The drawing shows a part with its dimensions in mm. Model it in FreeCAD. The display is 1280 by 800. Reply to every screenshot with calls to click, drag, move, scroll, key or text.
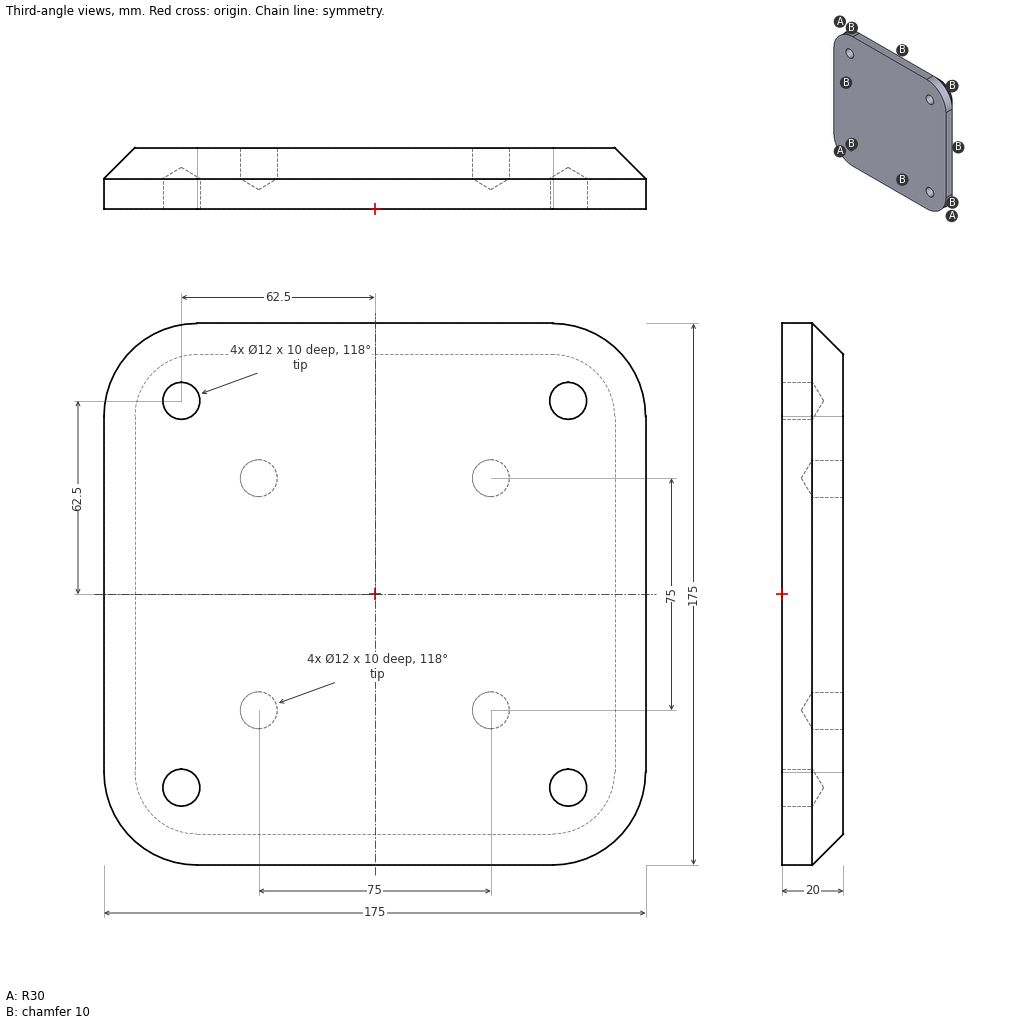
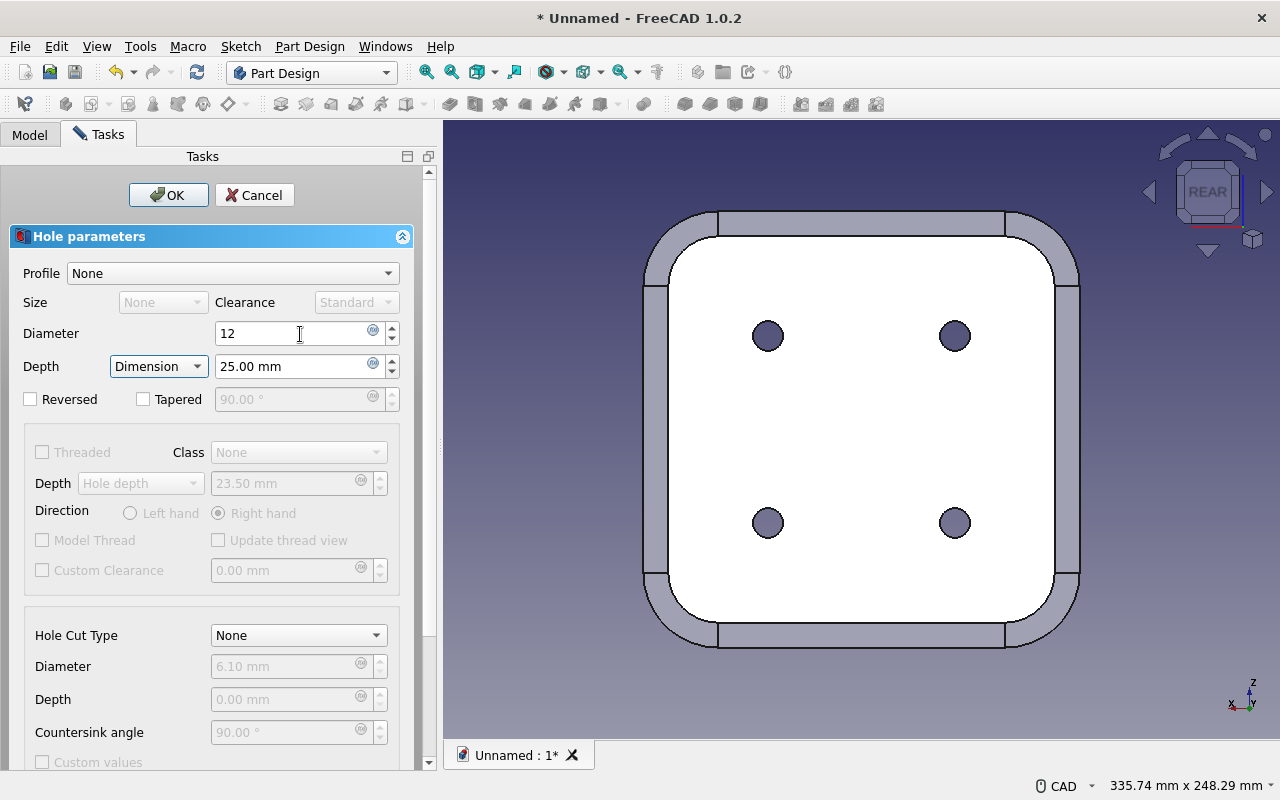
triple_click(300, 366)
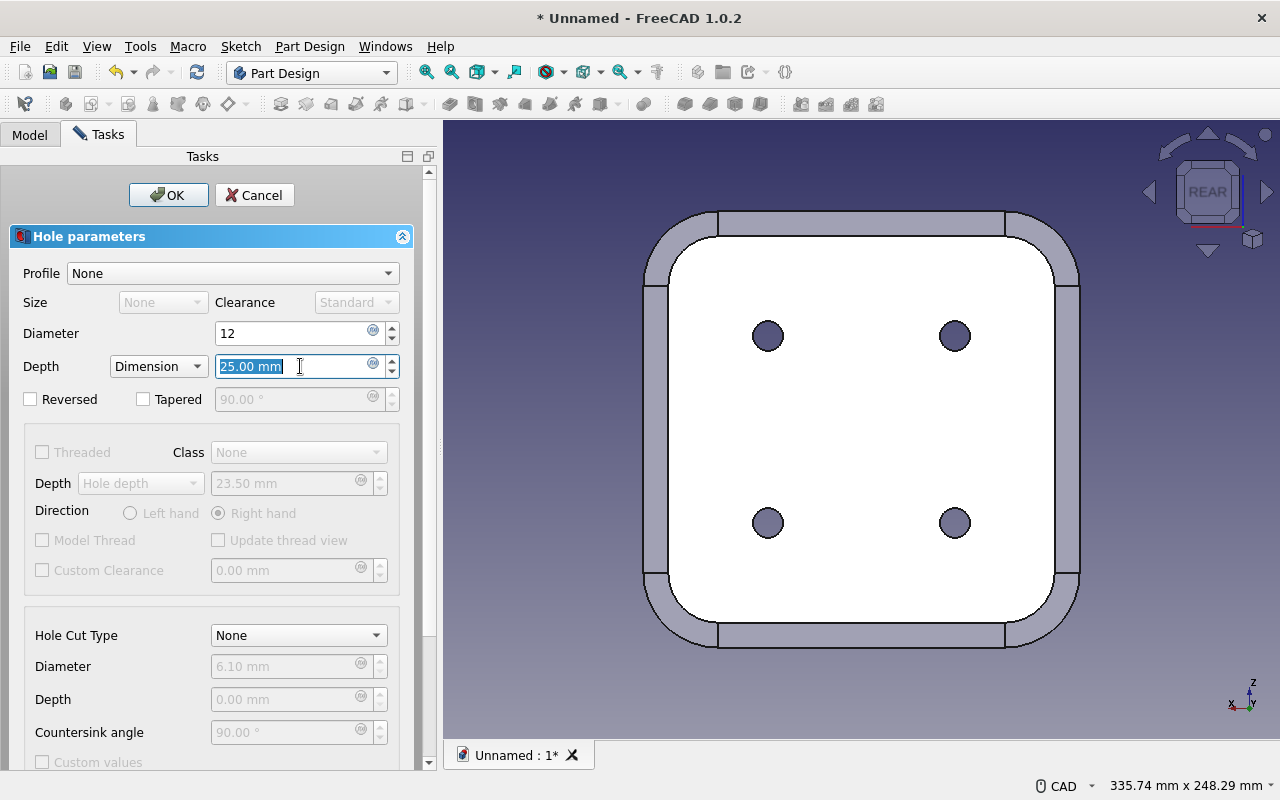
text(10)
key(Tab)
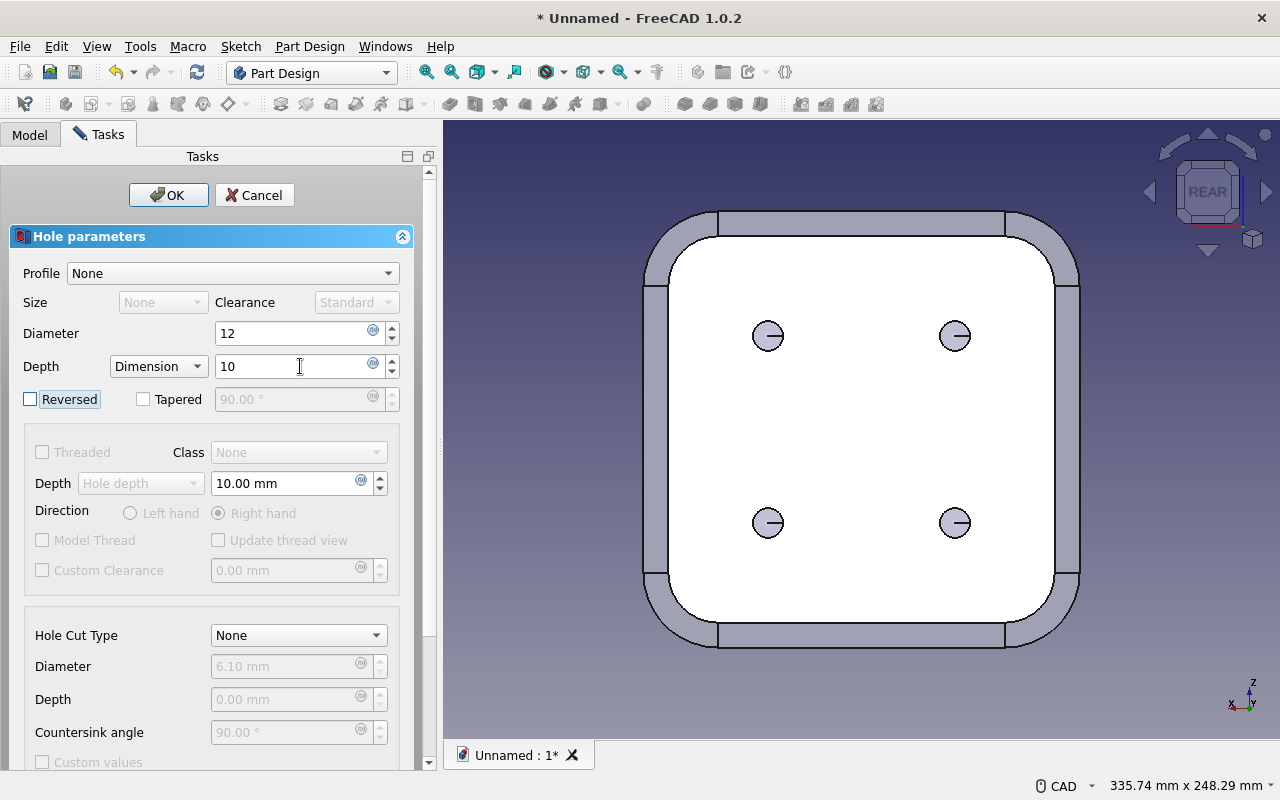
click(169, 195)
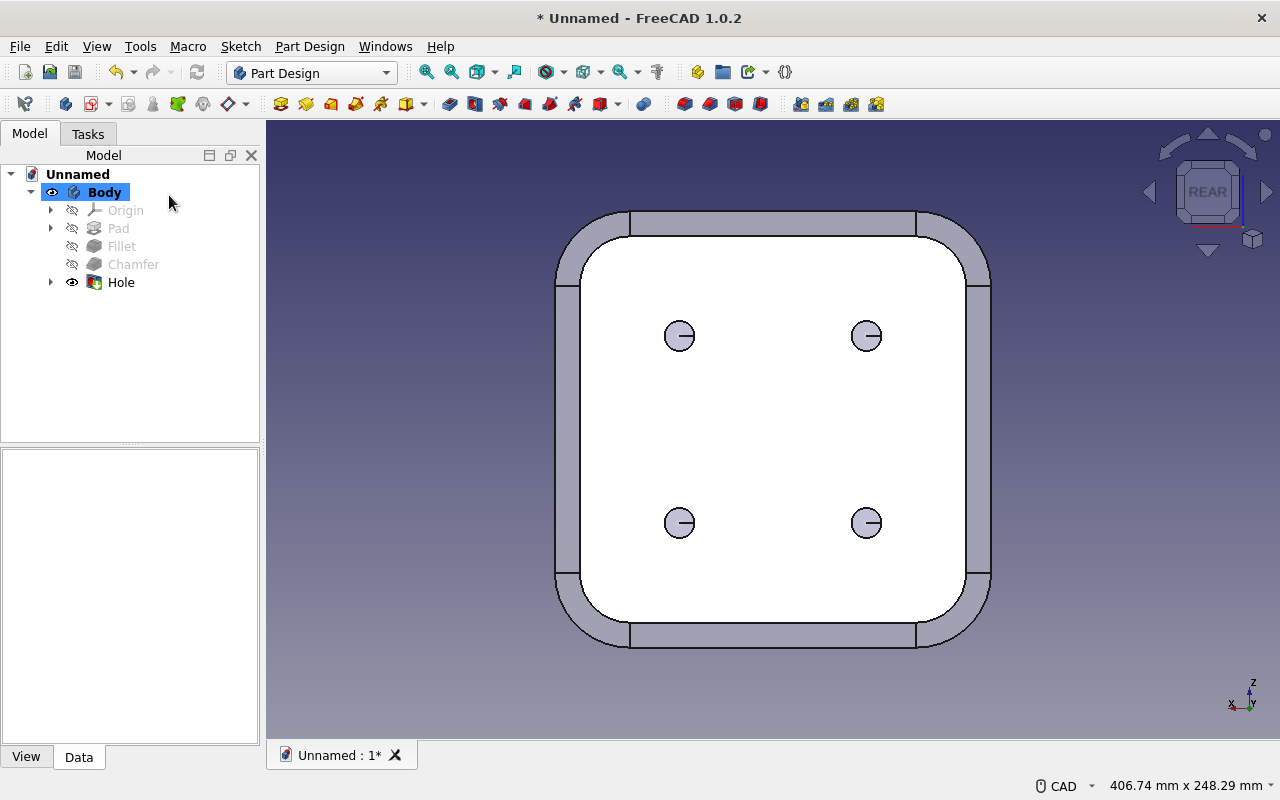
click(90, 104)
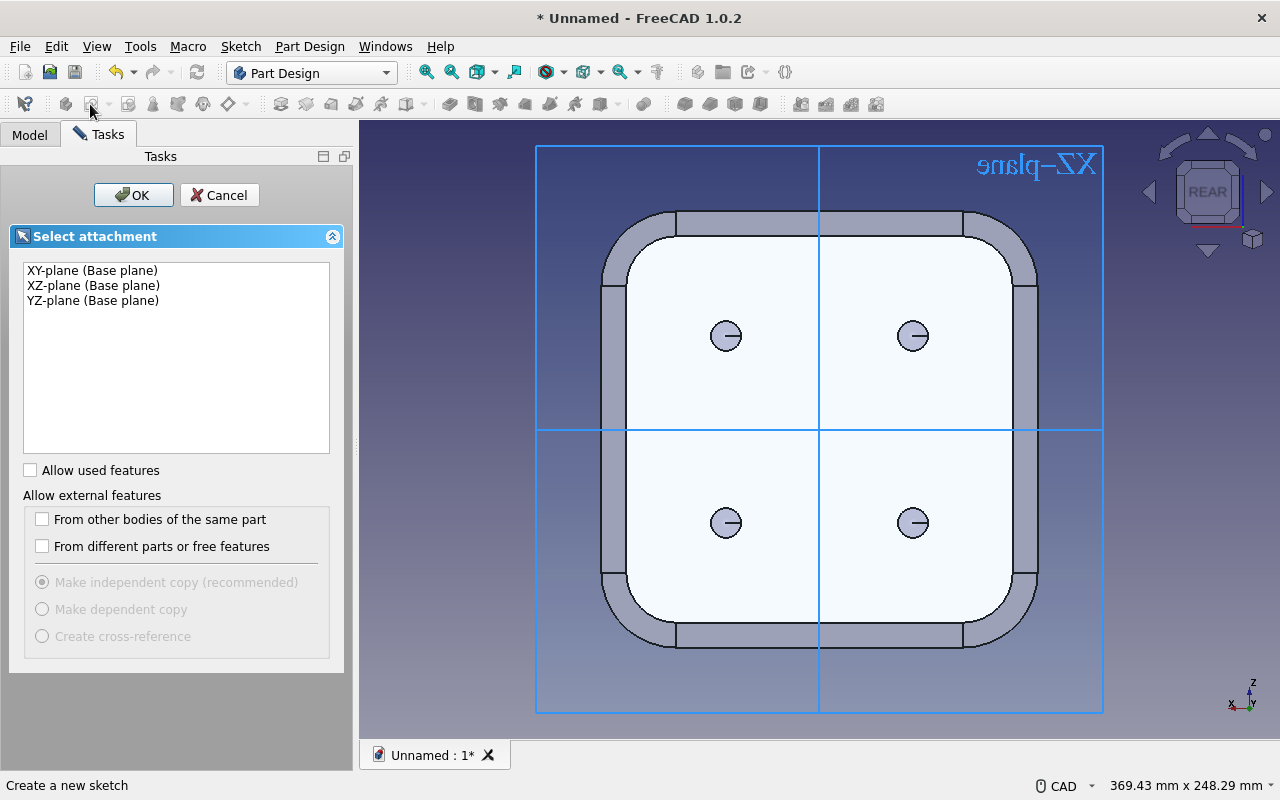
click(84, 286)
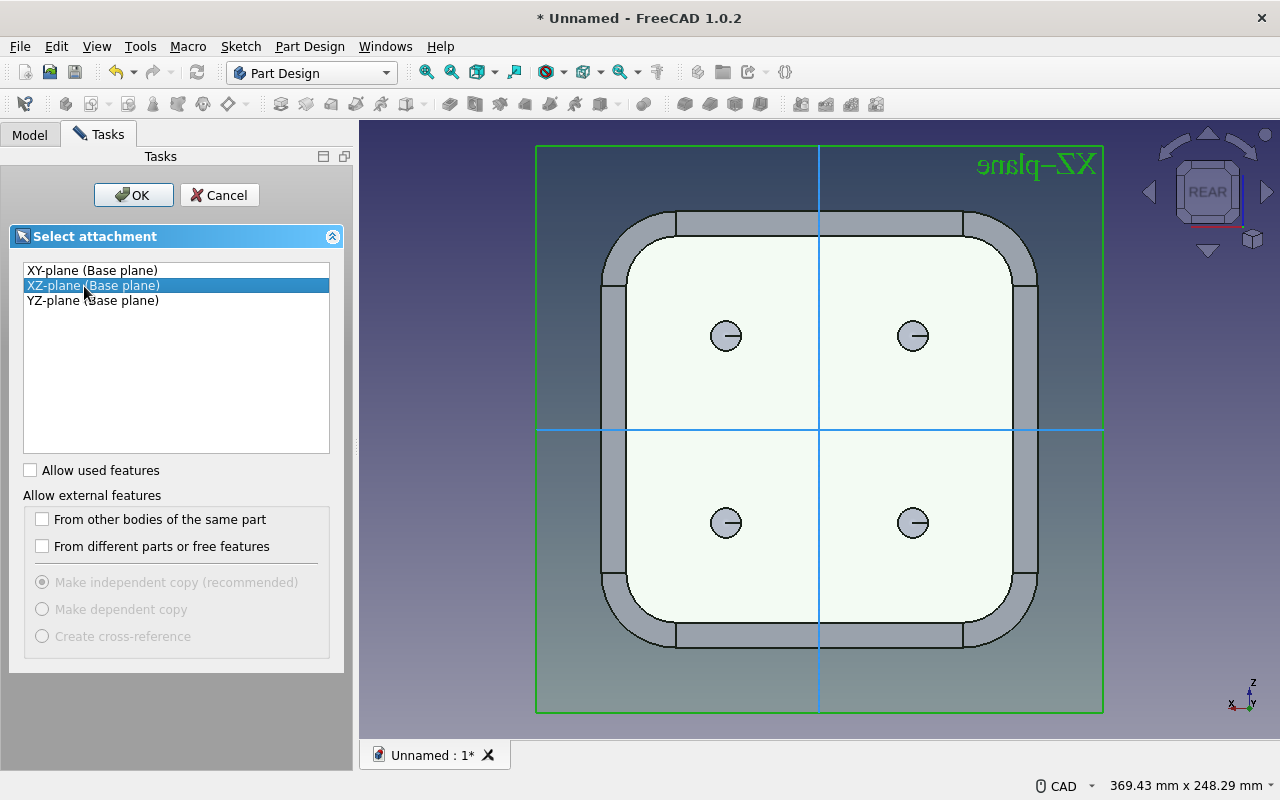
click(134, 195)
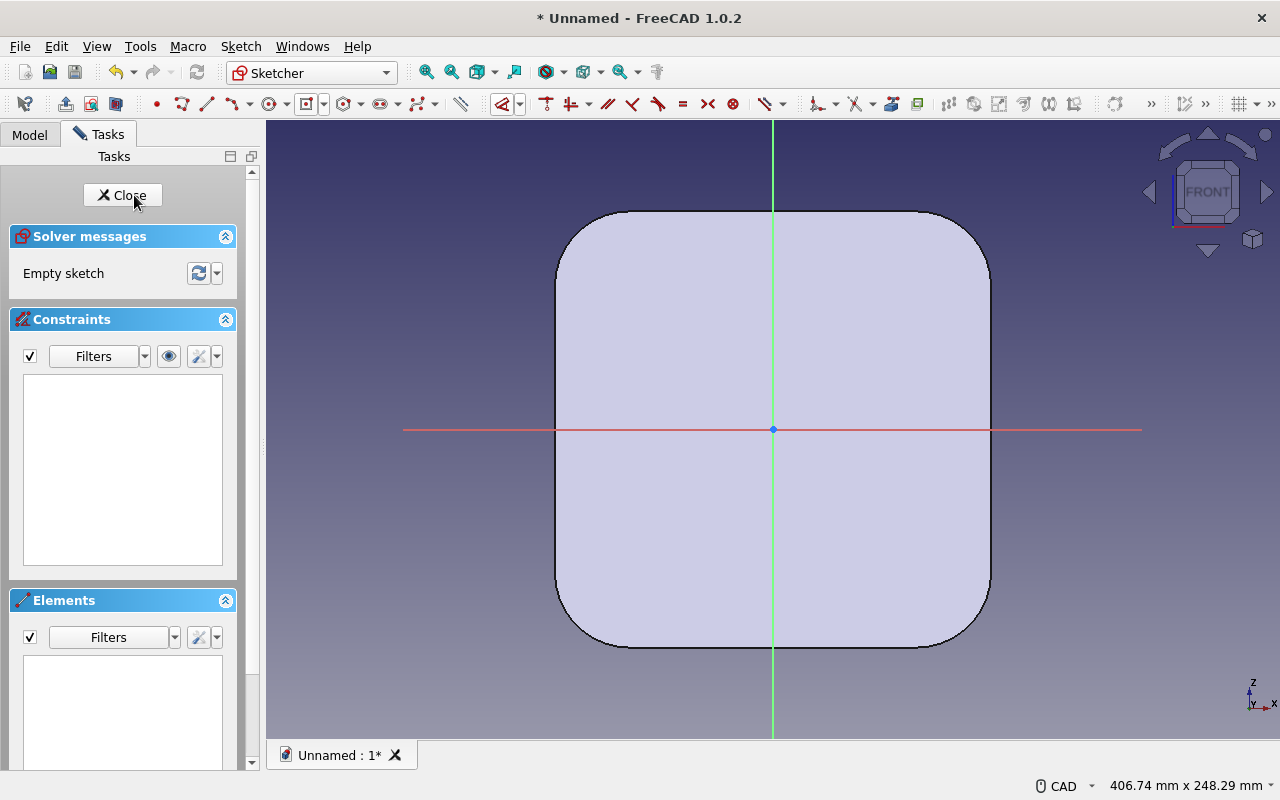
click(268, 104)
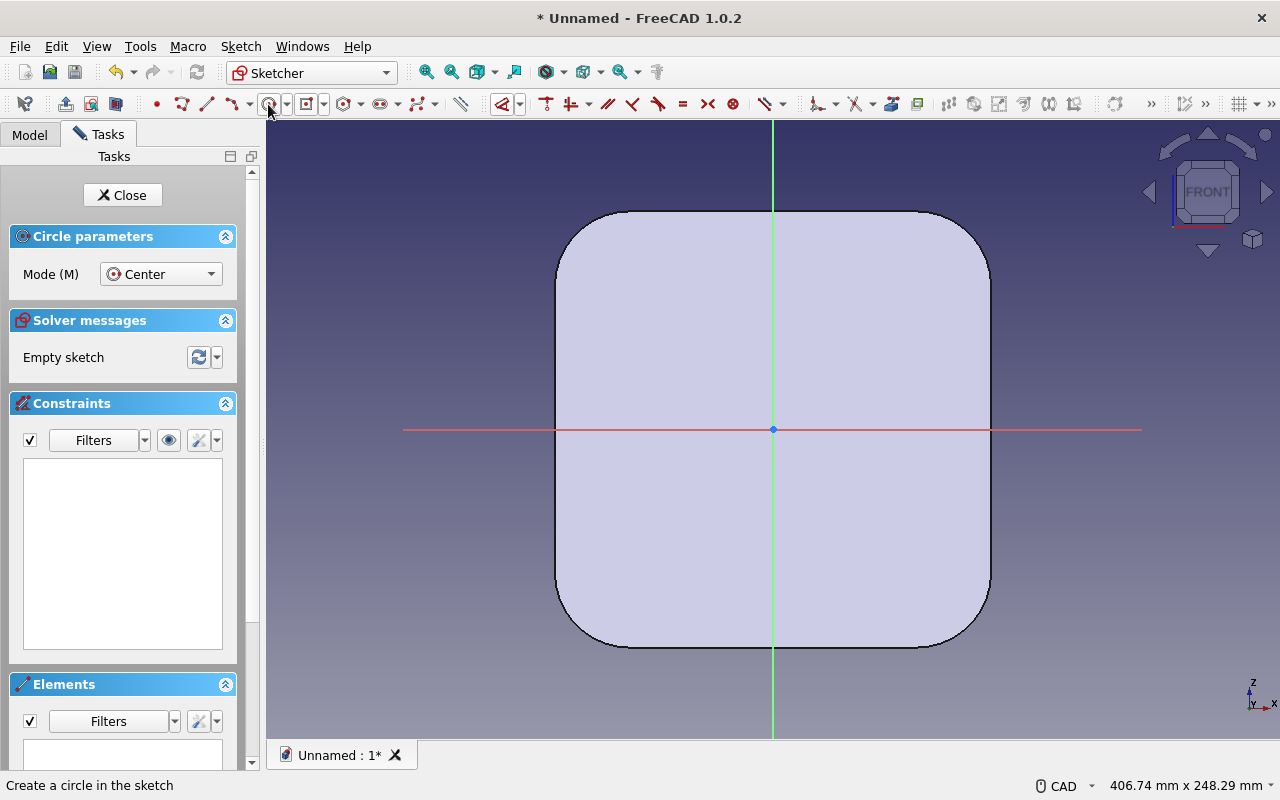
scroll(617, 274, up, 3)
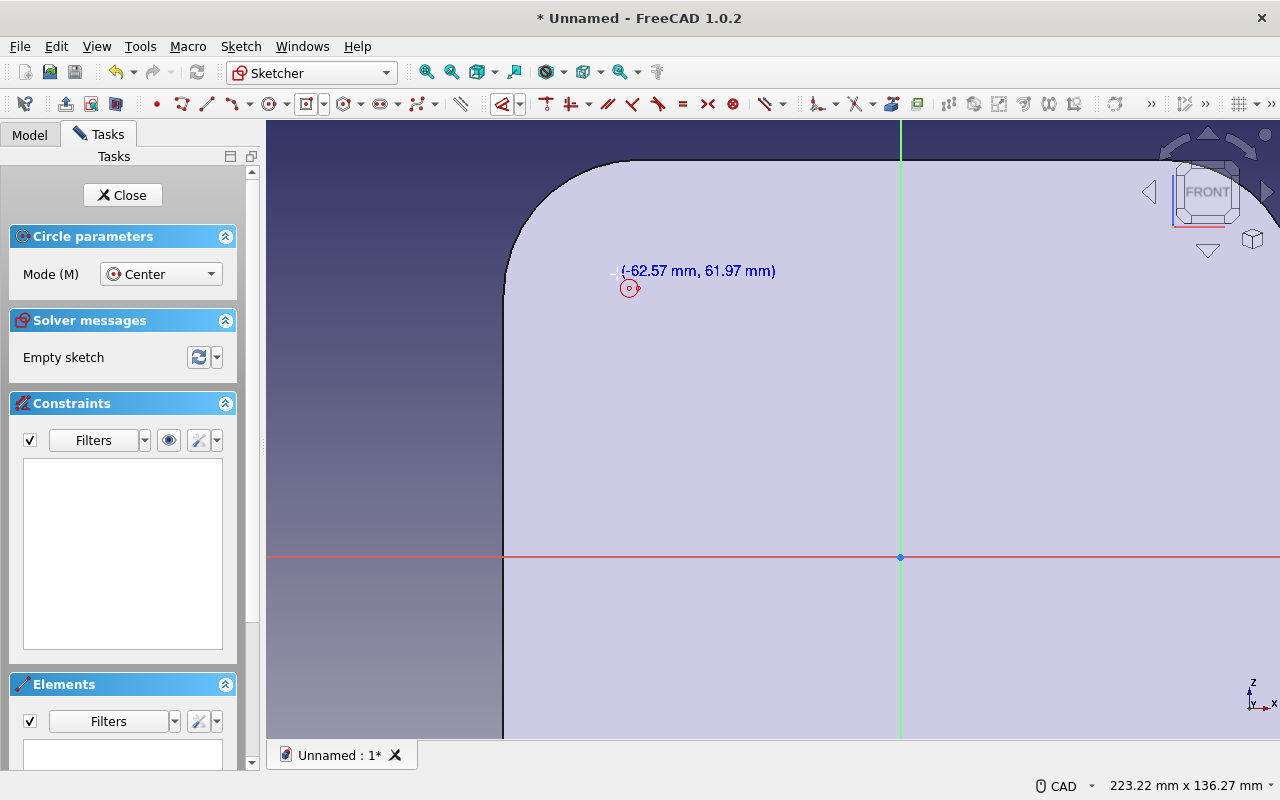
click(617, 273)
click(636, 254)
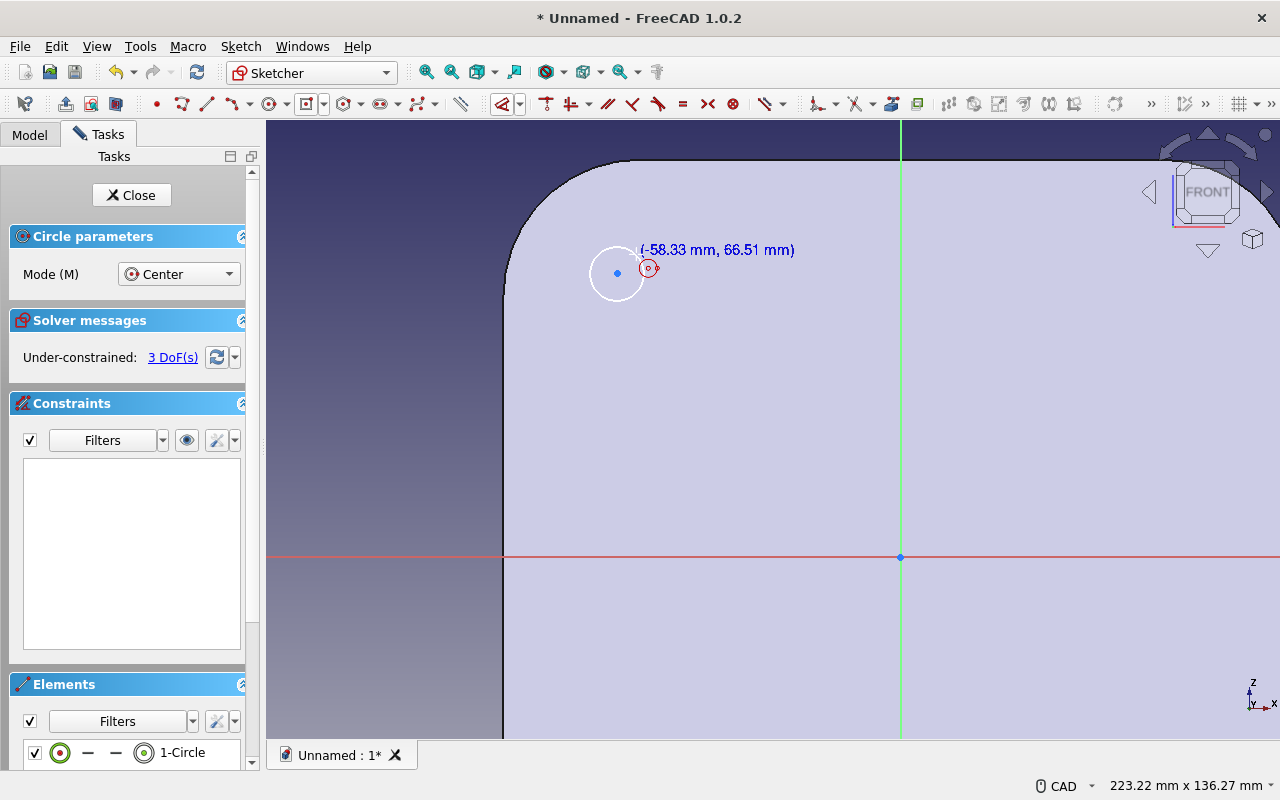
scroll(305, 170, down, 2)